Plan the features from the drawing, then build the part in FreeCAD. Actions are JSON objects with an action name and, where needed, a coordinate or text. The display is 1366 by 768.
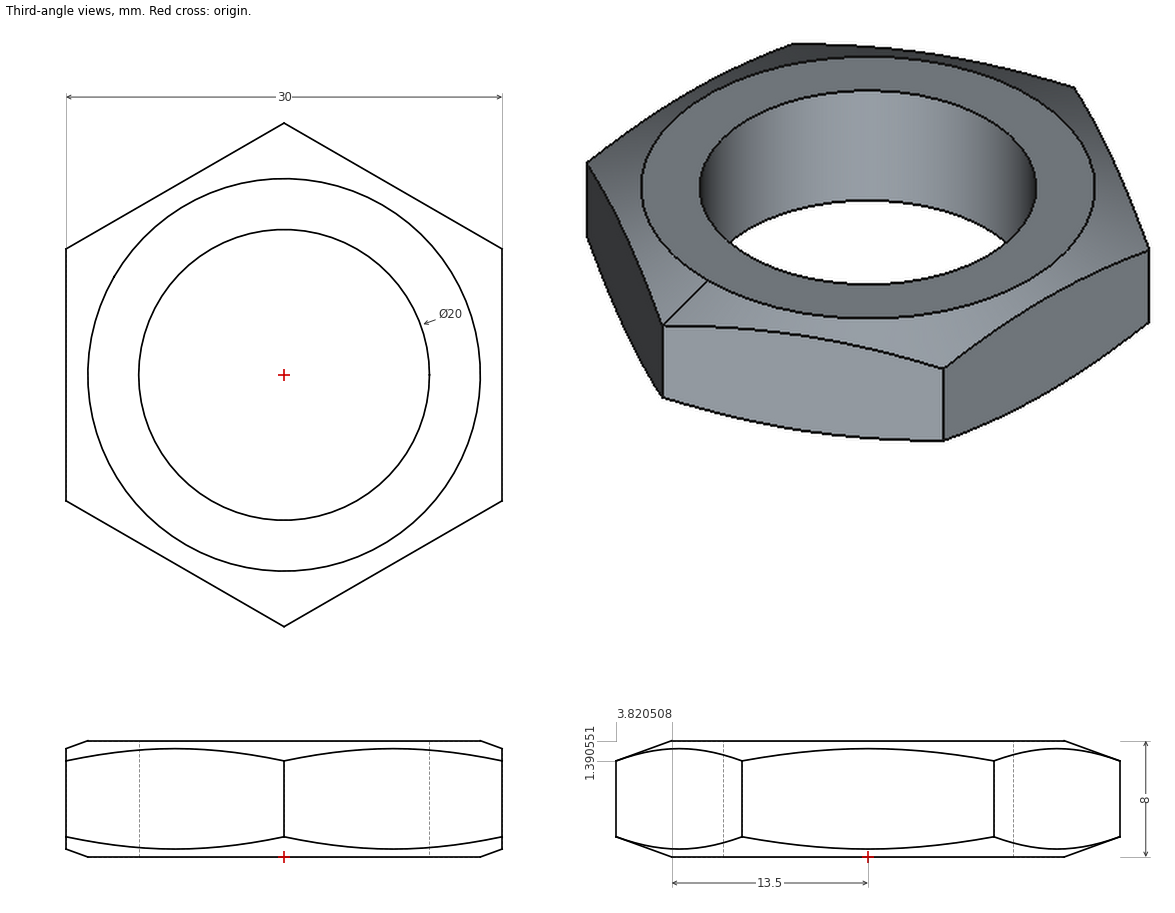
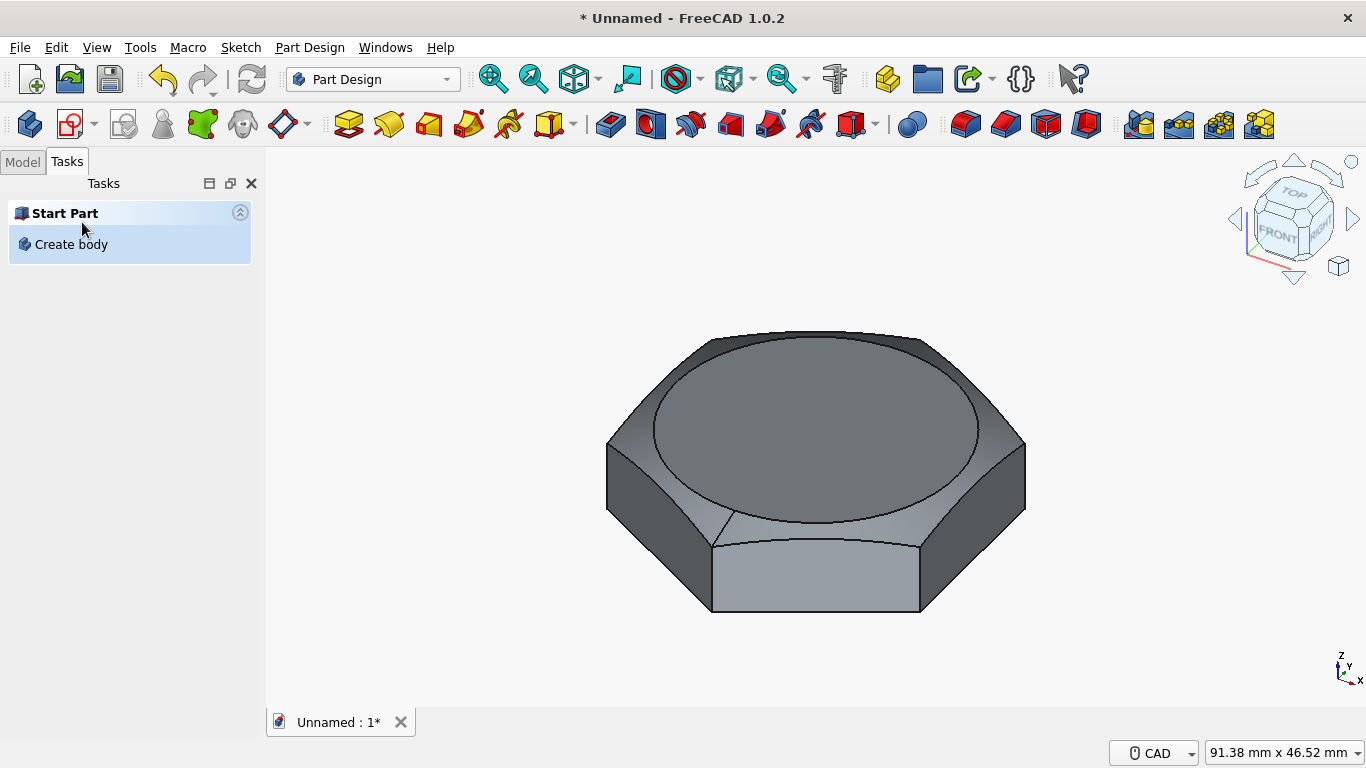
{"action": "left_click", "coordinate": [23, 161]}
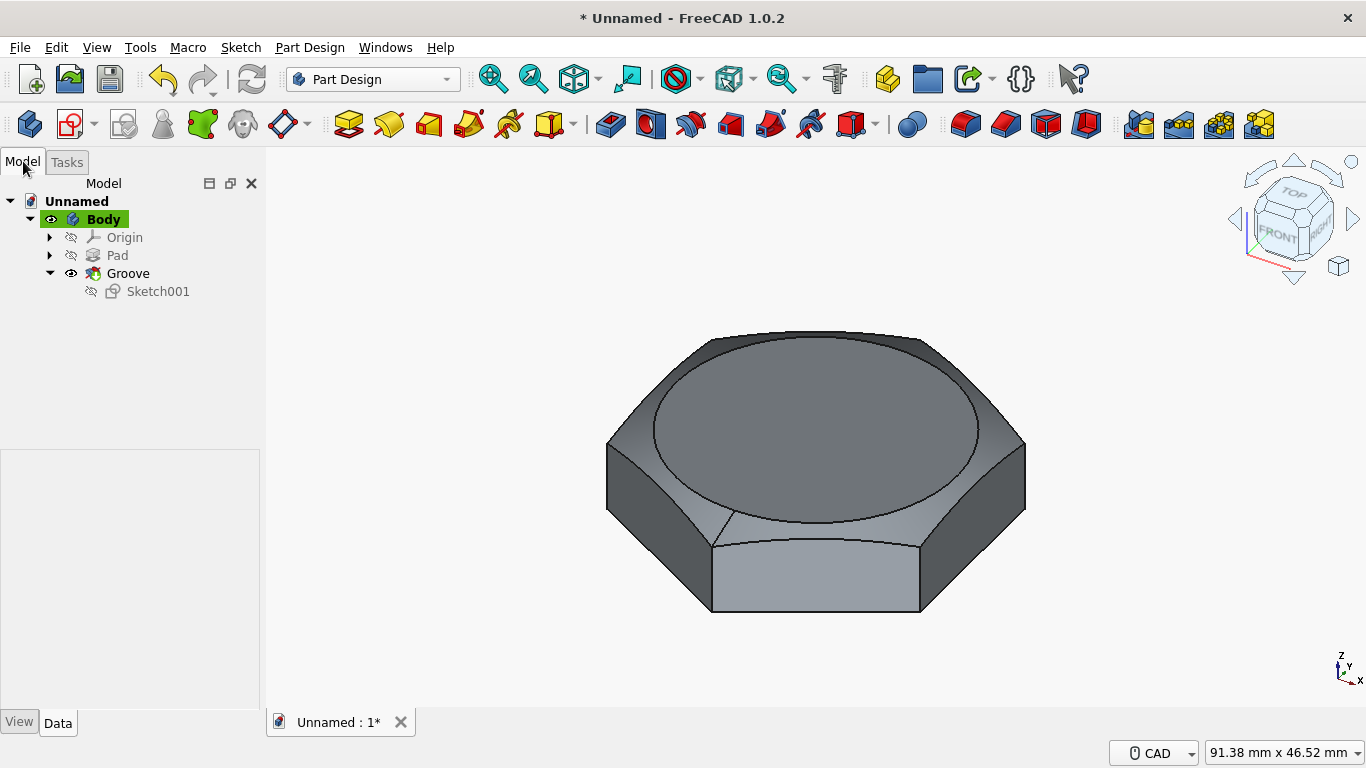
{"action": "left_click", "coordinate": [50, 237]}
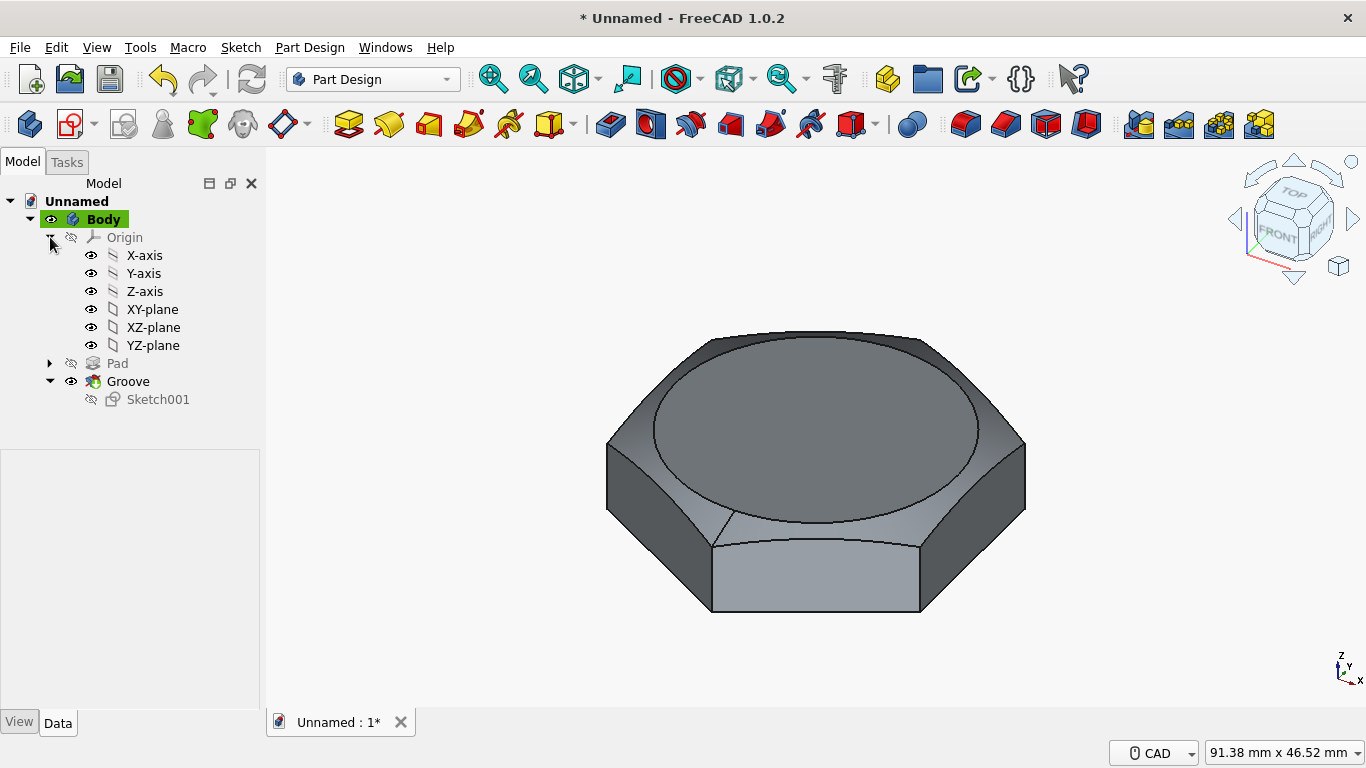
{"action": "left_click", "coordinate": [136, 309]}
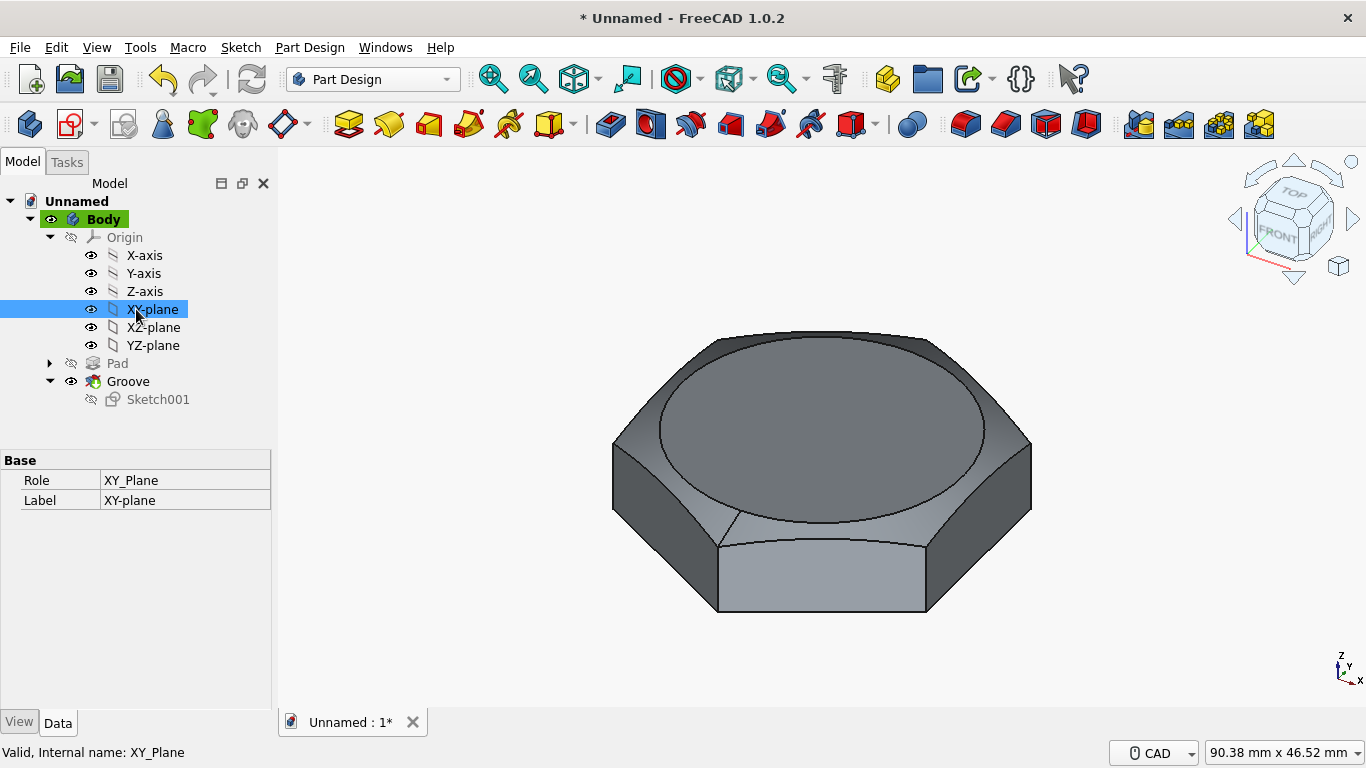
{"action": "left_click", "coordinate": [284, 124]}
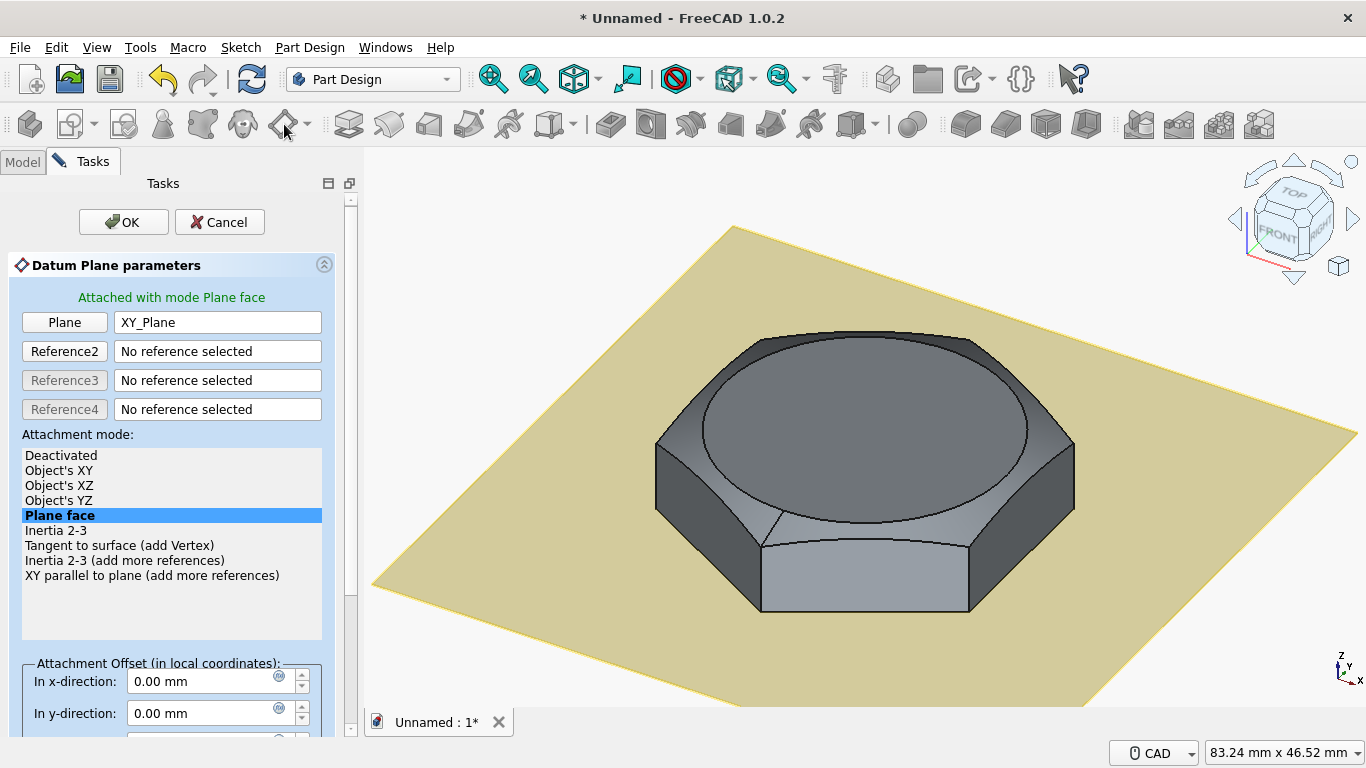
{"action": "scroll", "coordinate": [351, 464], "scroll_direction": "down", "scroll_amount": 2}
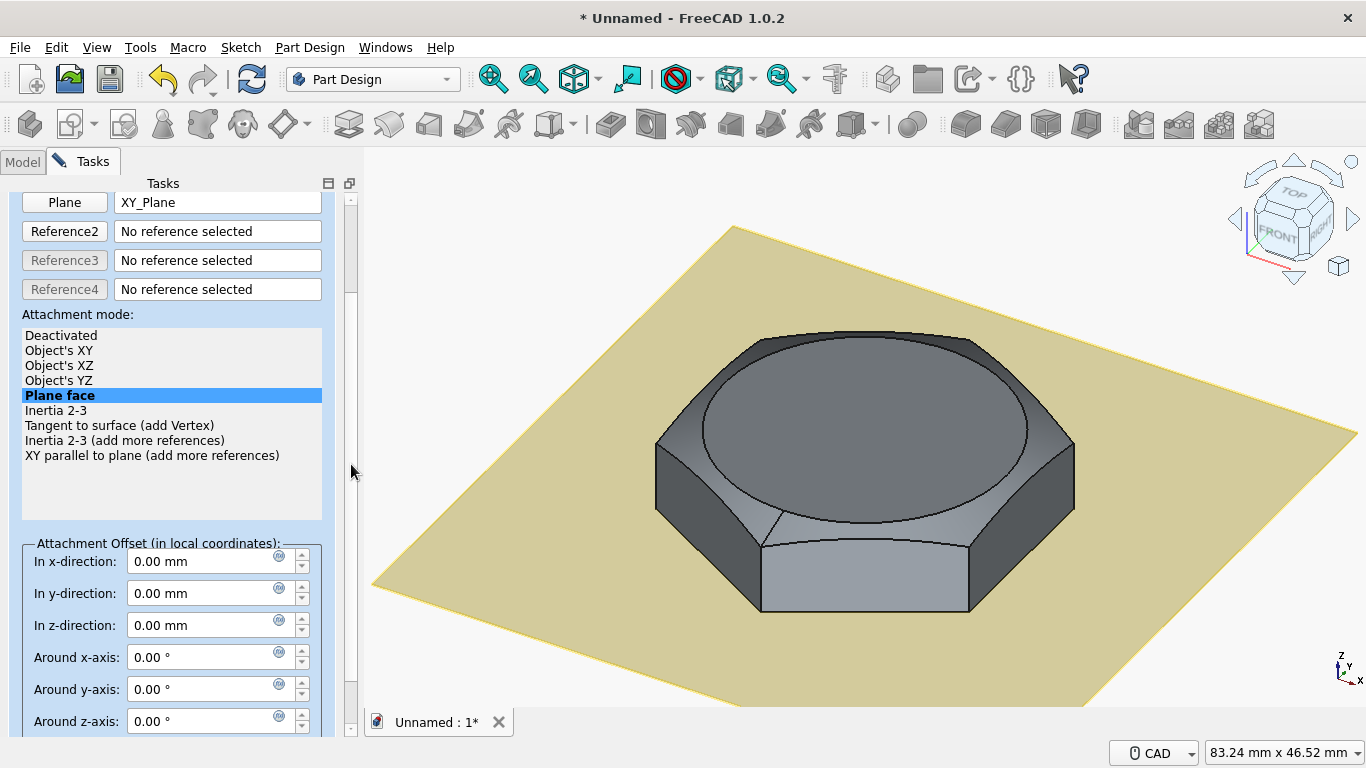
{"action": "triple_click", "coordinate": [210, 625]}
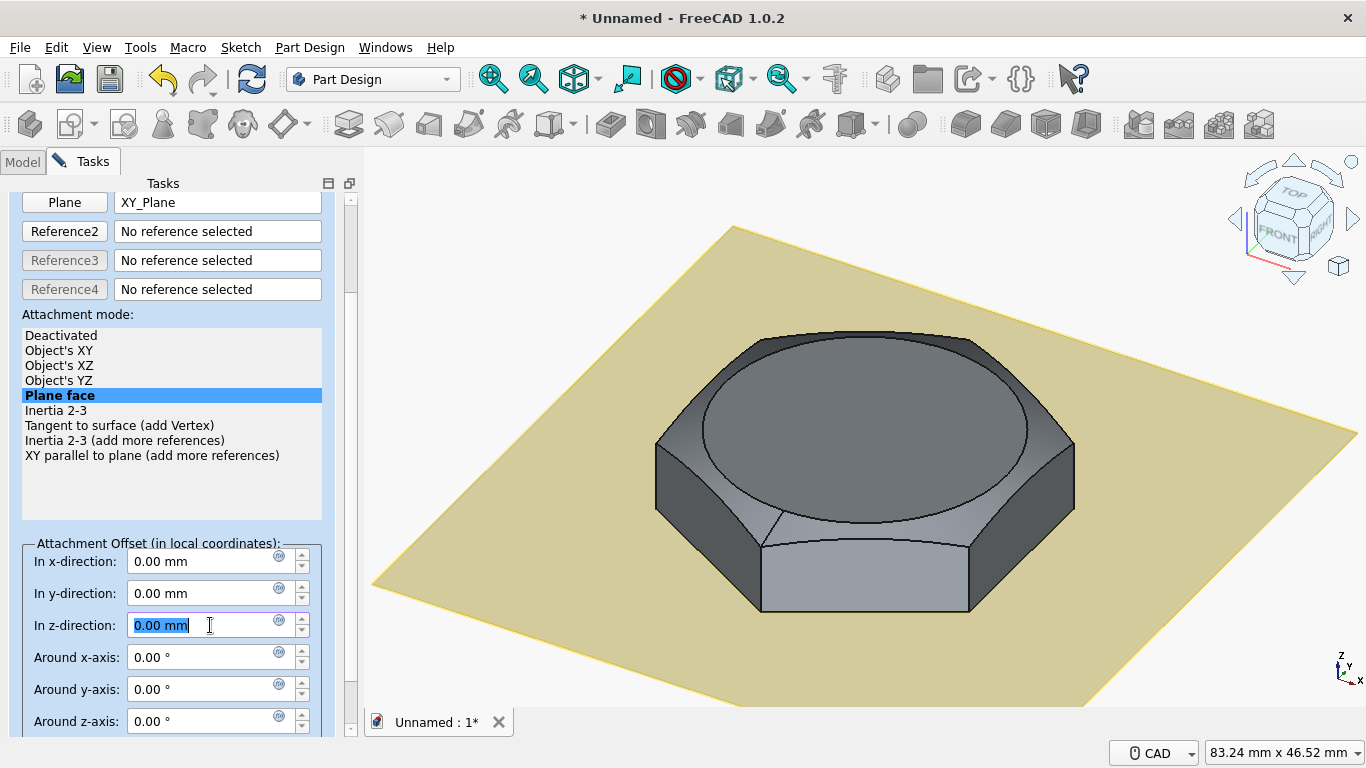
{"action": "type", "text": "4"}
{"action": "key", "text": "Tab"}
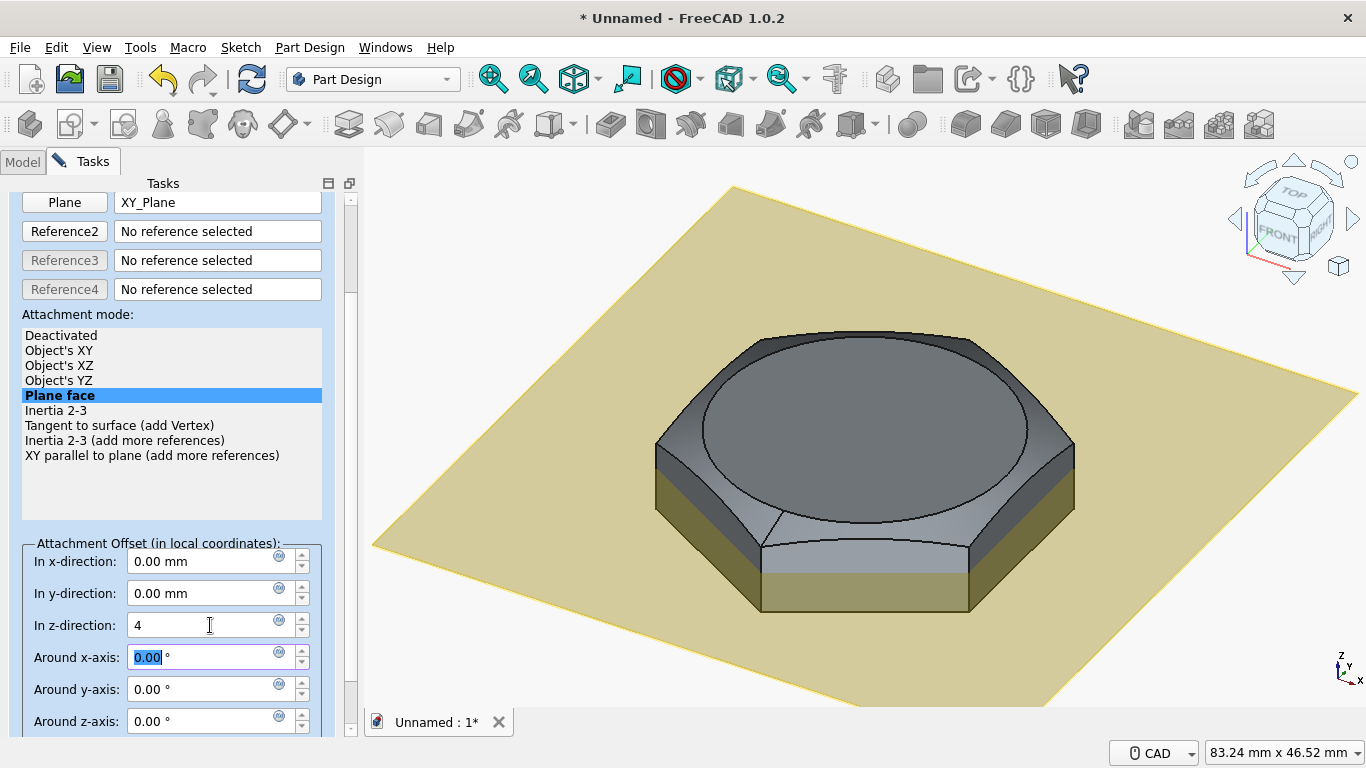
{"action": "scroll", "coordinate": [351, 464], "scroll_direction": "up", "scroll_amount": 3}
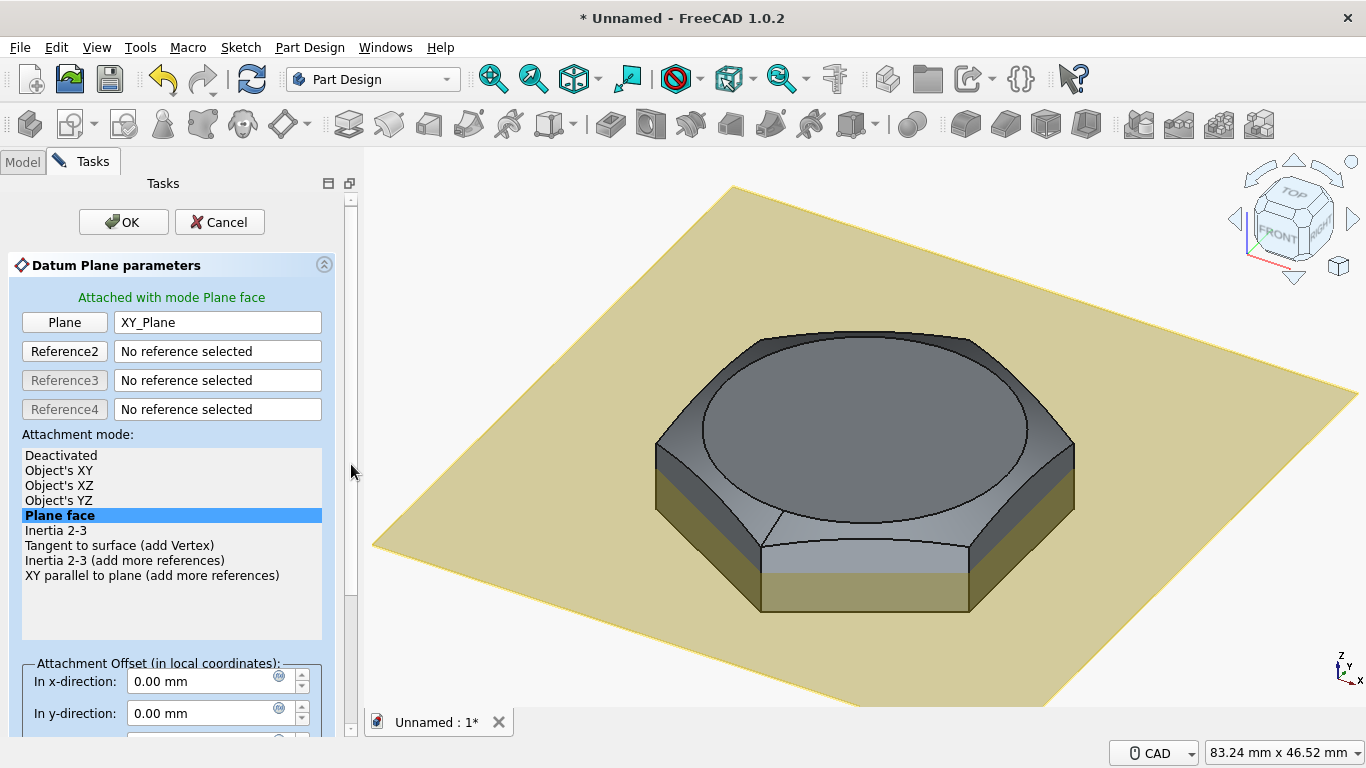
{"action": "left_click", "coordinate": [124, 222]}